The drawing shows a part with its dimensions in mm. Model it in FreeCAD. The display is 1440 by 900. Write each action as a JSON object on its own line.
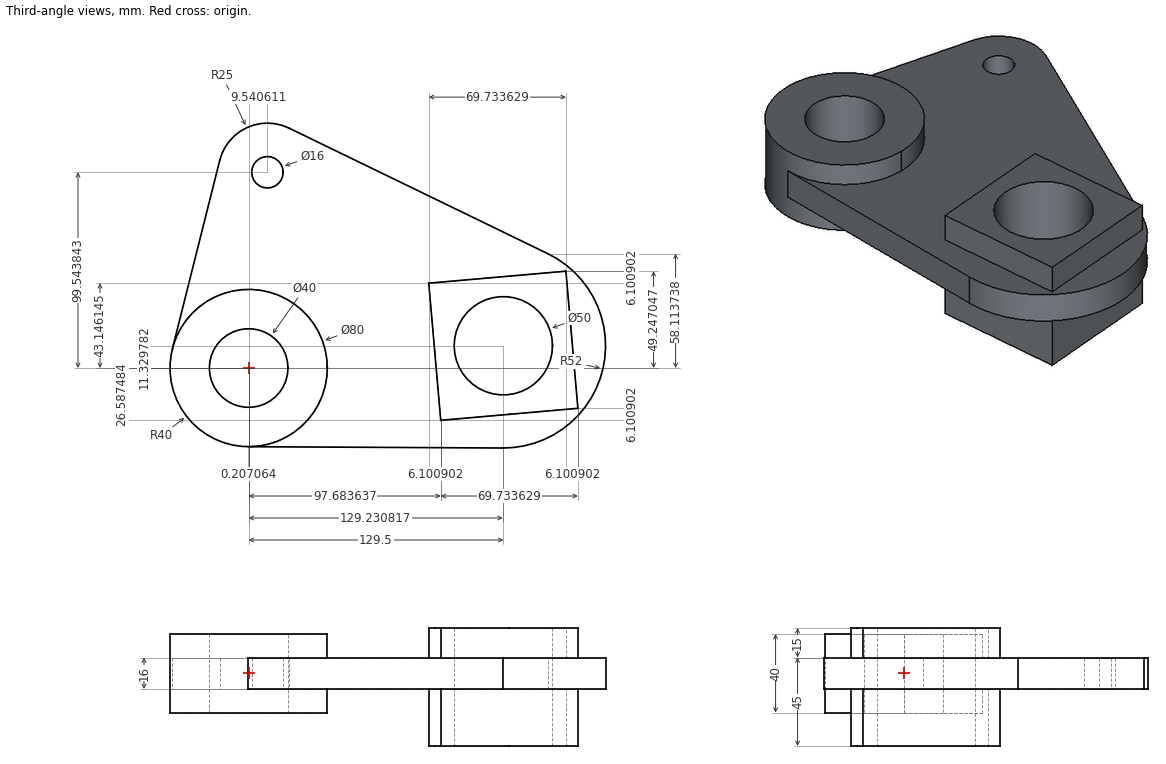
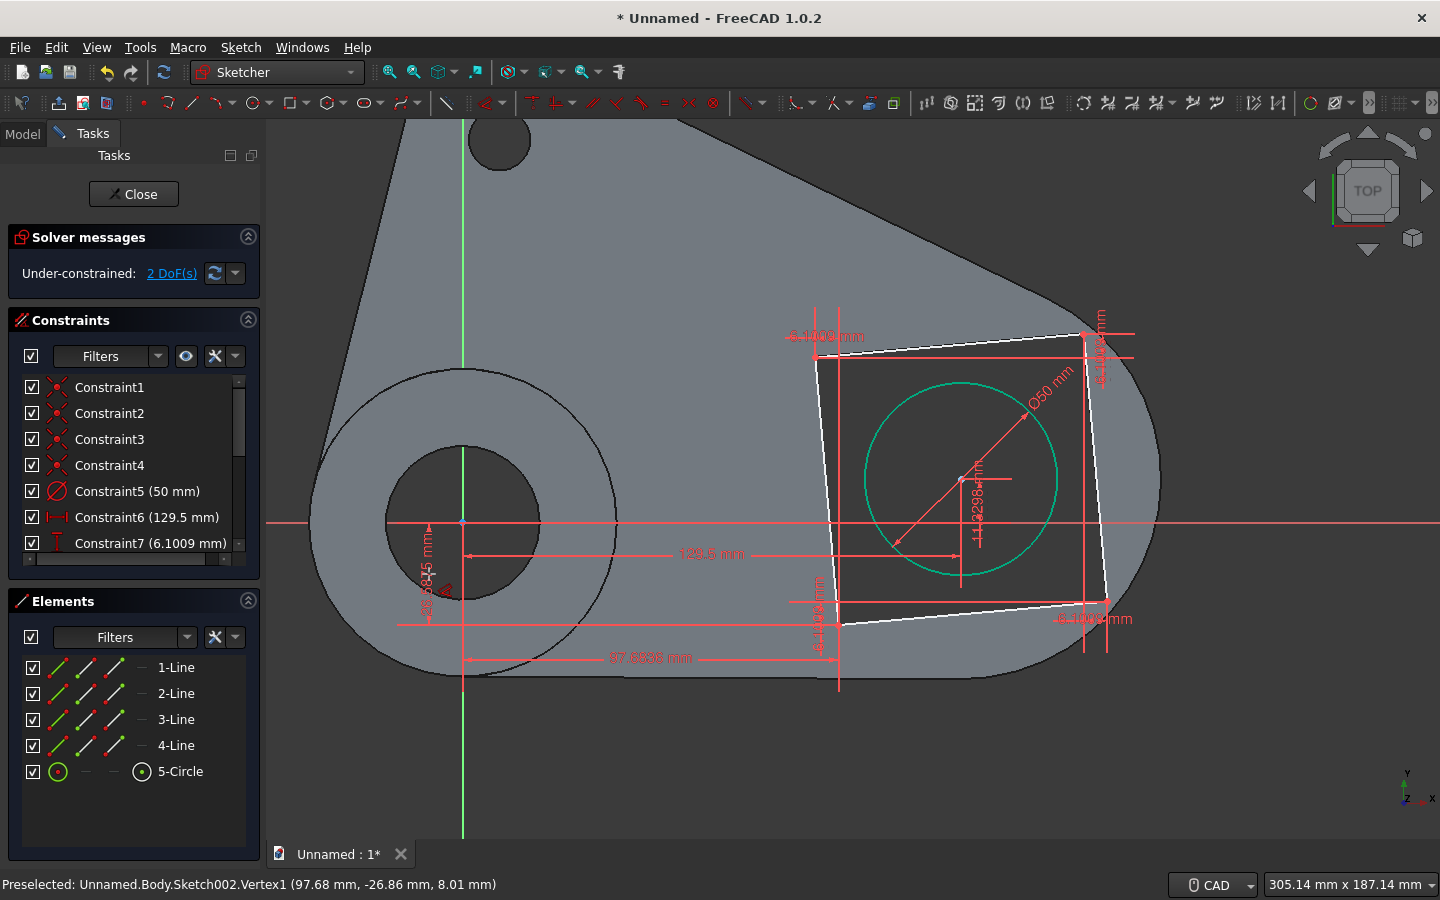
{"action": "left_click", "coordinate": [1084, 334]}
{"action": "left_click", "coordinate": [429, 428]}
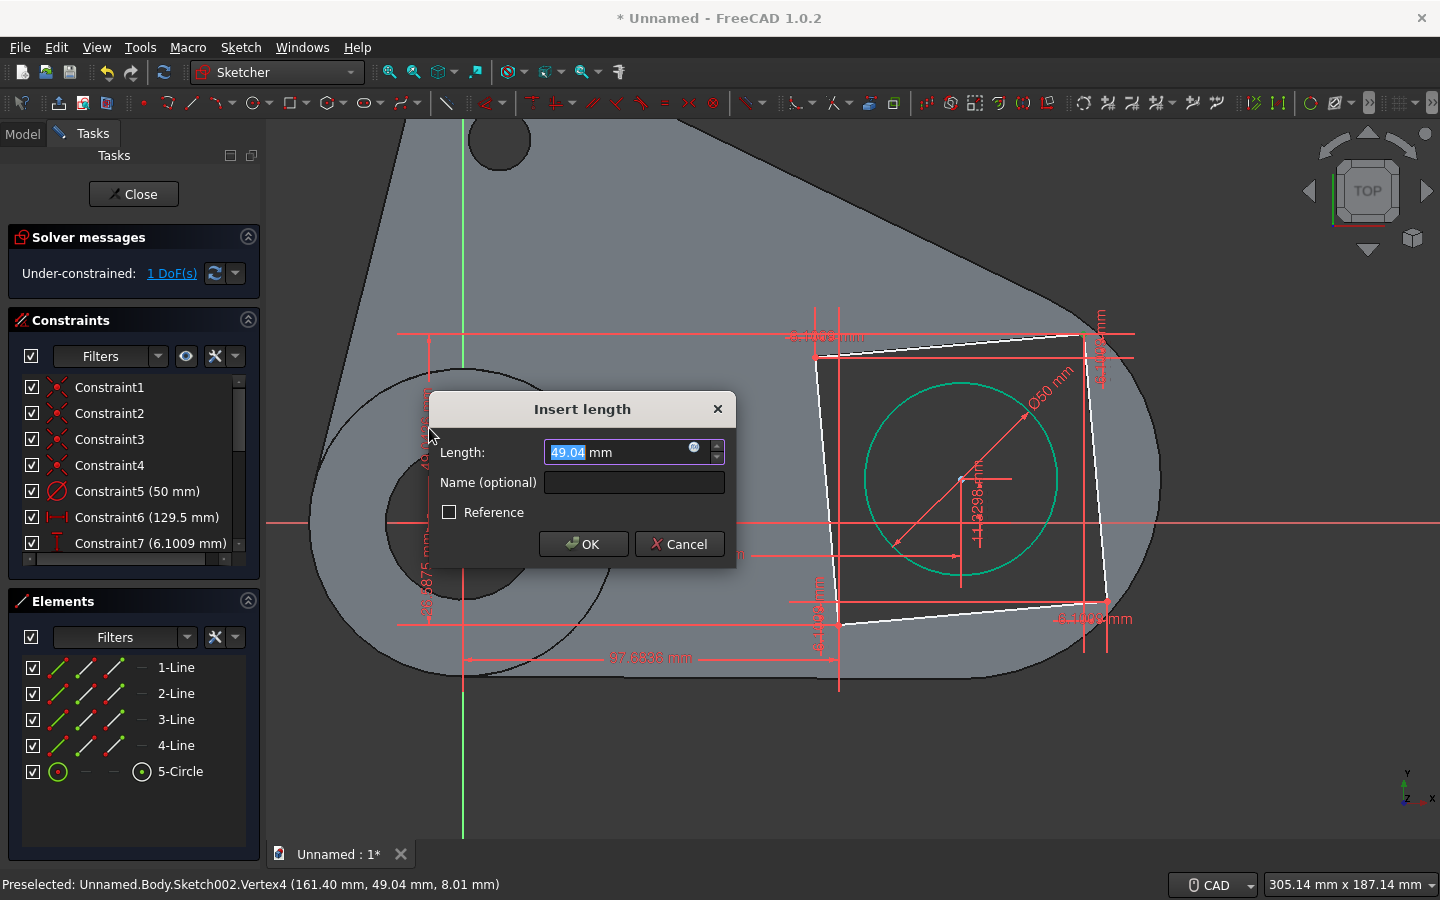
{"action": "type", "text": "49.247047"}
{"action": "key", "text": "Return"}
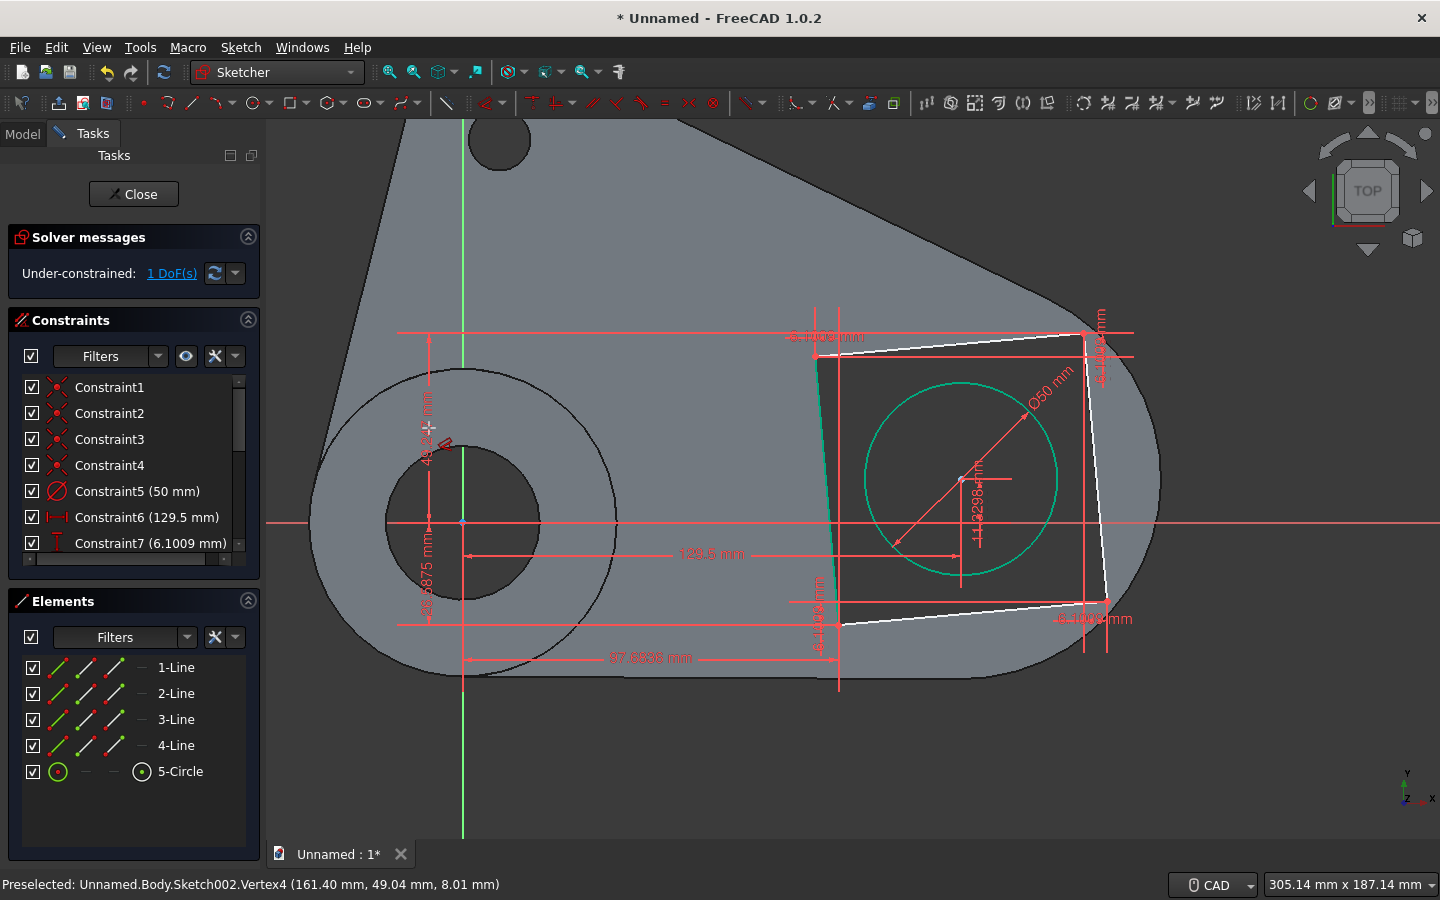
{"action": "left_click", "coordinate": [919, 618]}
{"action": "left_click", "coordinate": [973, 659]}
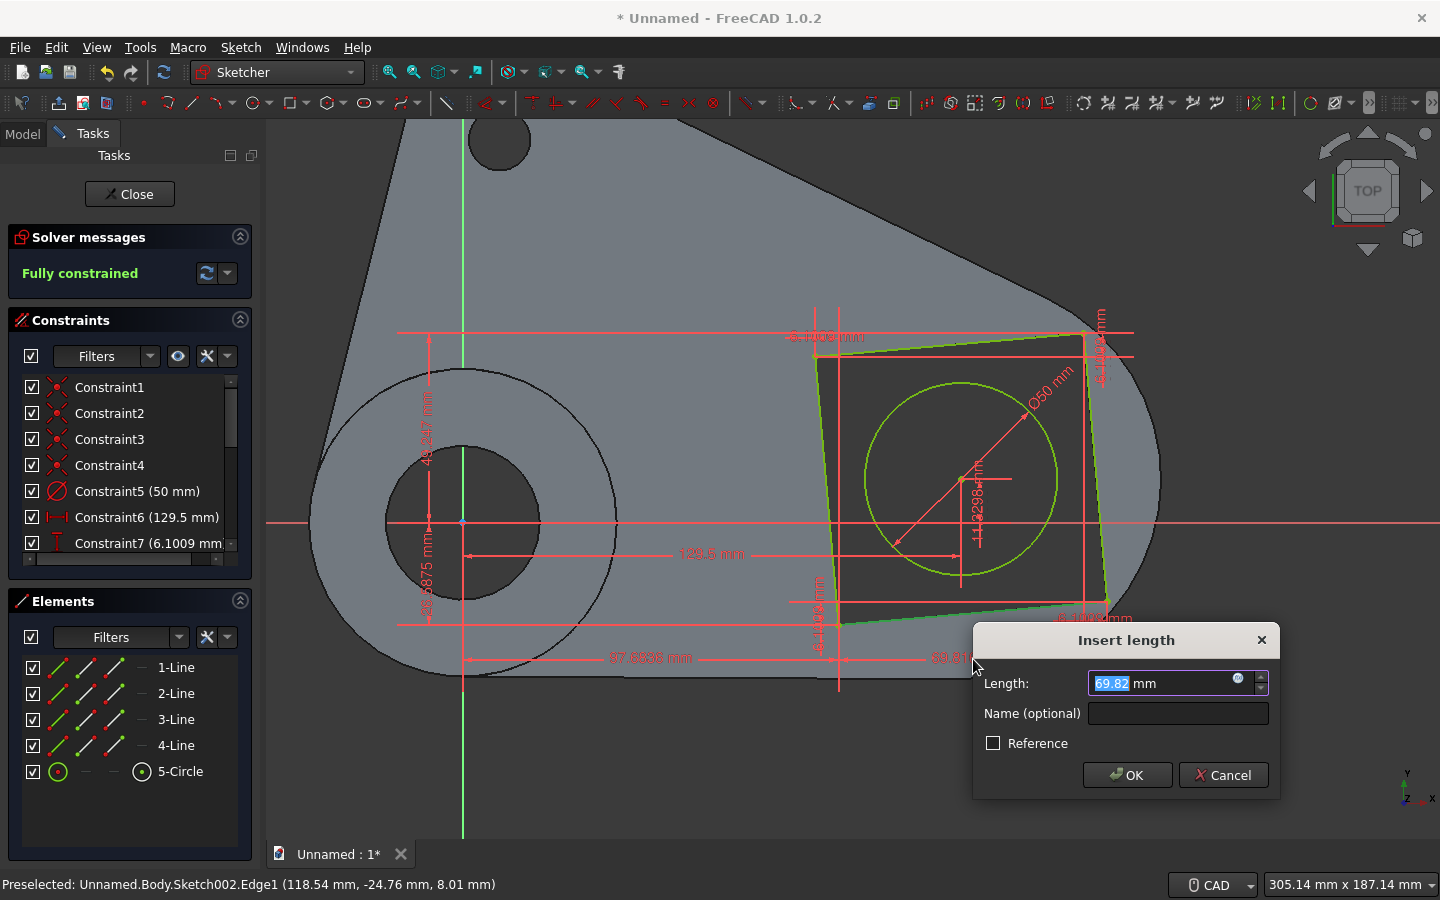
{"action": "type", "text": "69.733629"}
{"action": "key", "text": "Return"}
{"action": "key", "text": "Escape"}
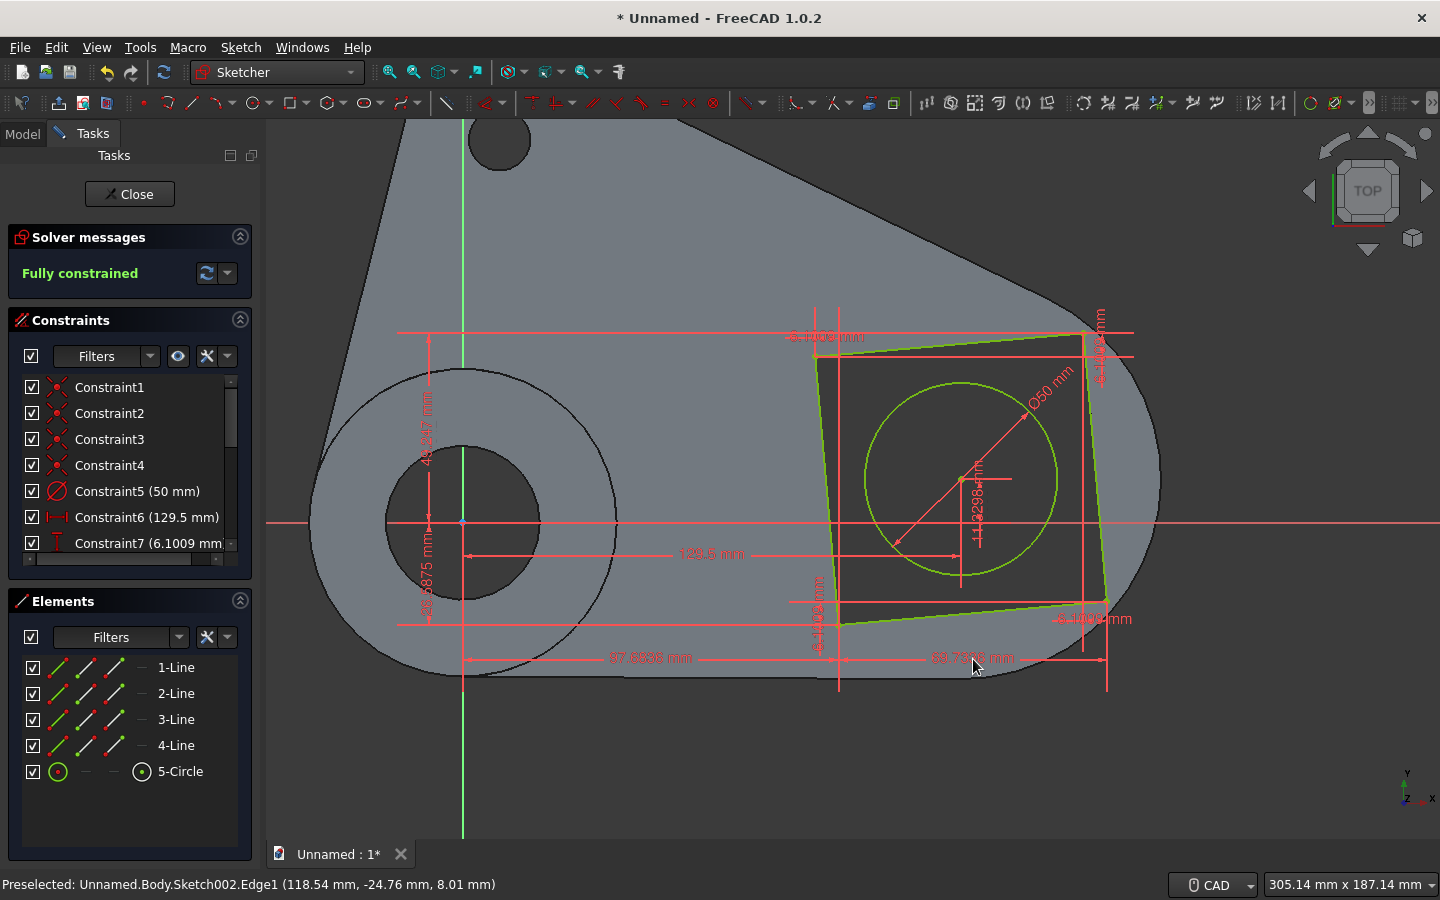
{"action": "left_click", "coordinate": [130, 194]}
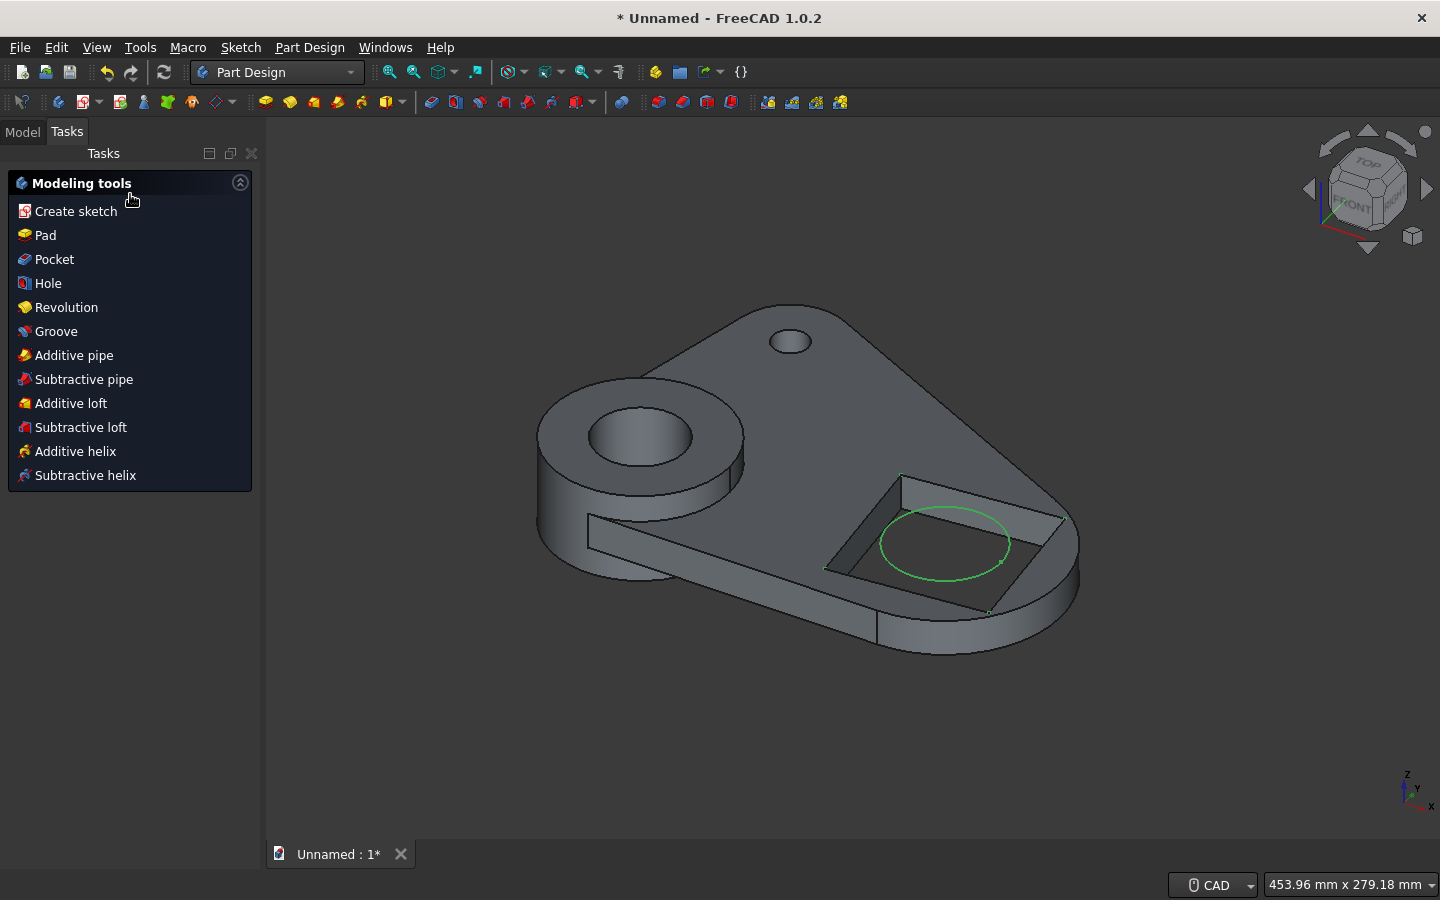
{"action": "left_click", "coordinate": [266, 102]}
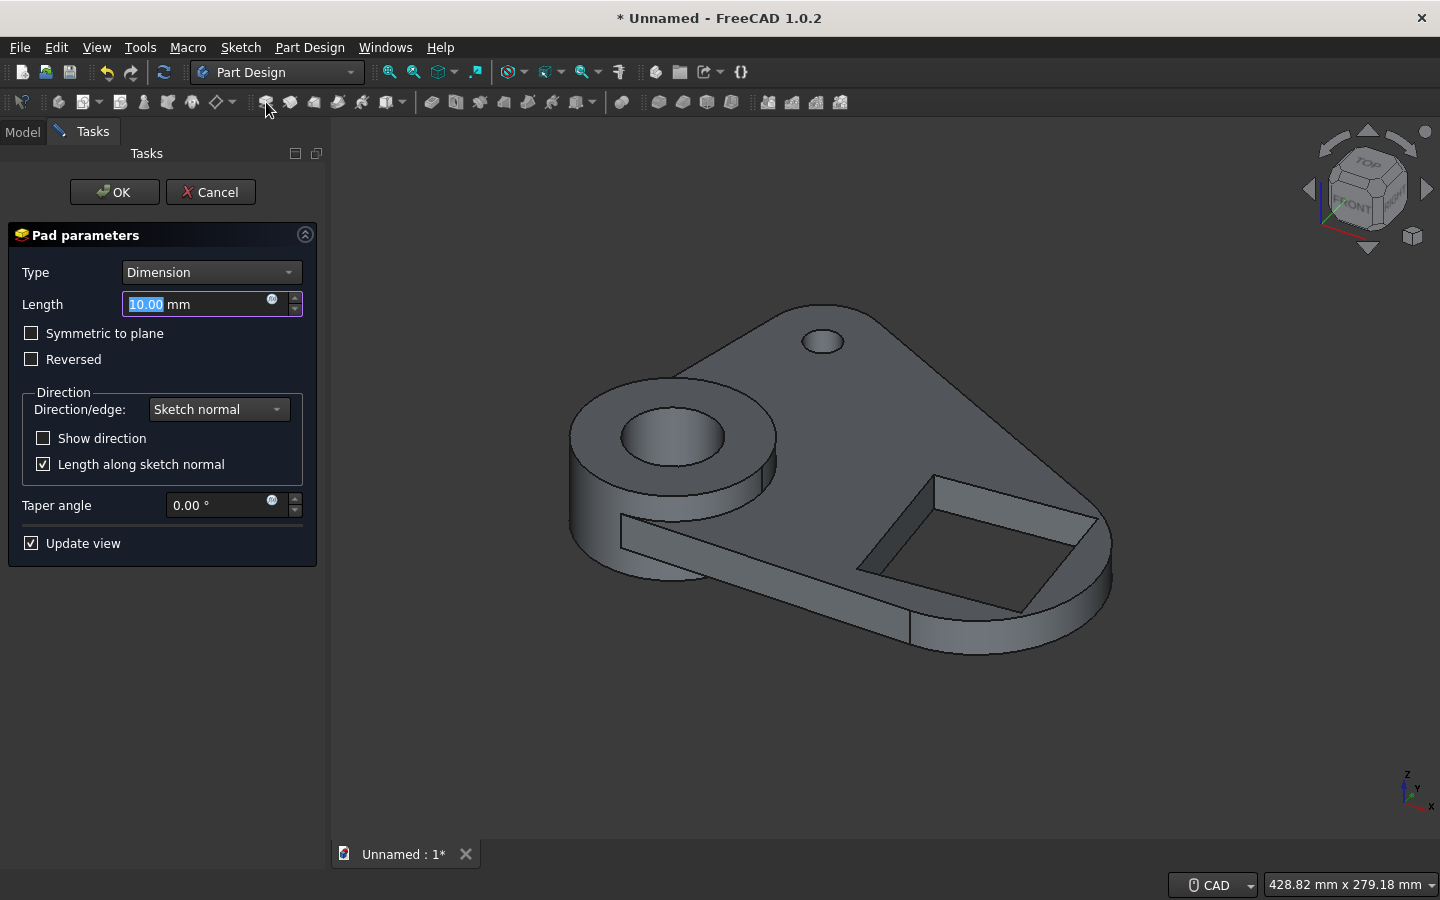
{"action": "left_click", "coordinate": [212, 272]}